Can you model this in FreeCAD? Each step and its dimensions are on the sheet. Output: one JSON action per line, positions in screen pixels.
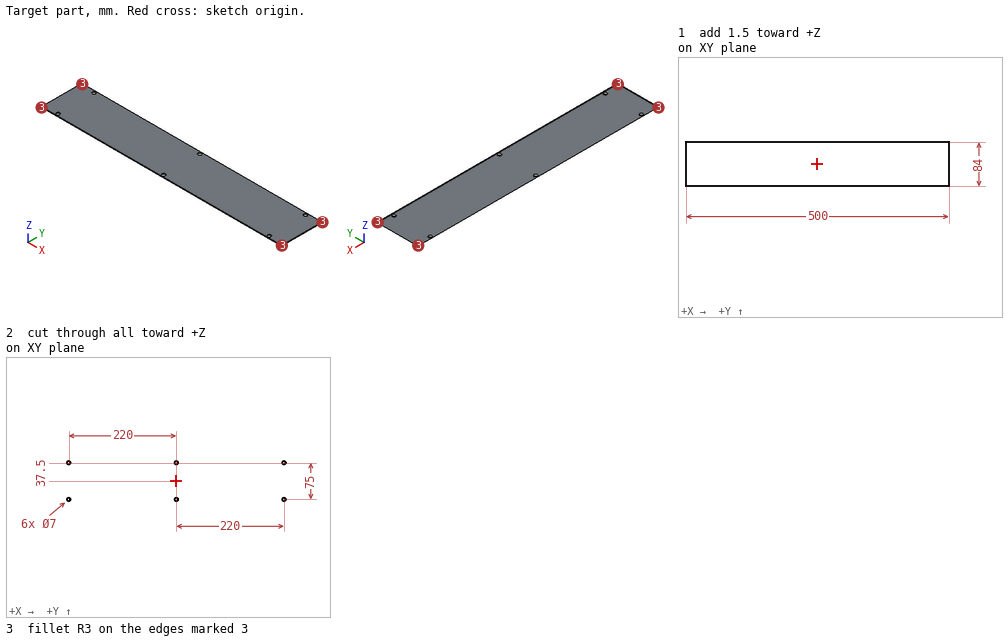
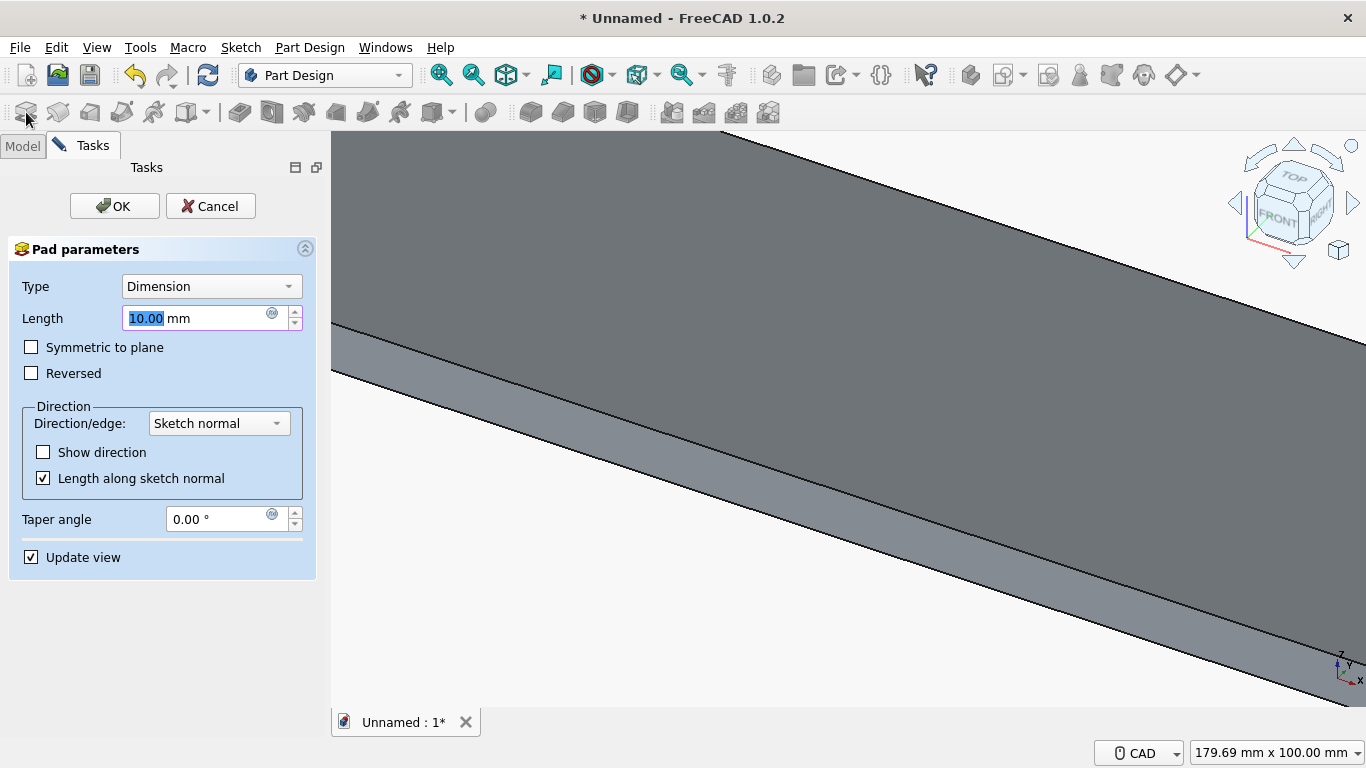
{"action": "type", "text": "1.5"}
{"action": "key", "text": "Tab"}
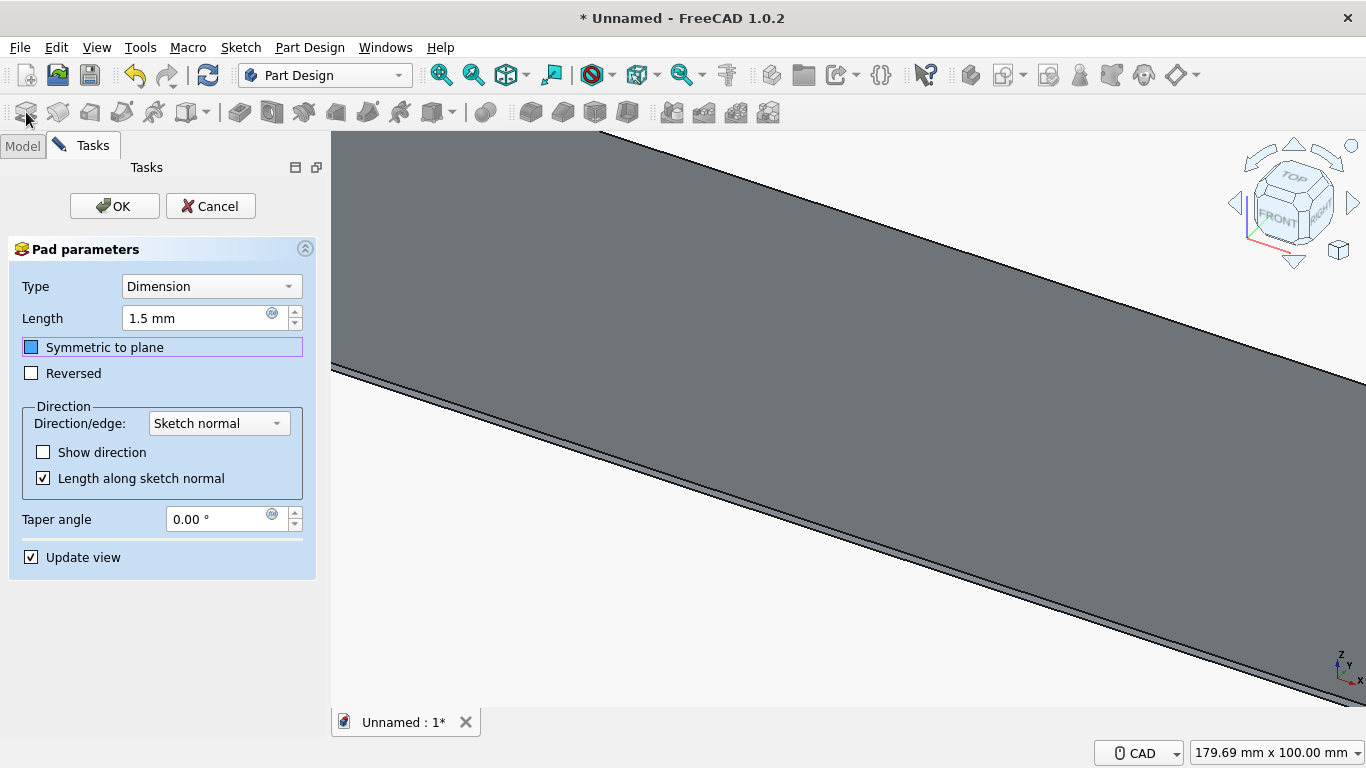
{"action": "left_click", "coordinate": [115, 206]}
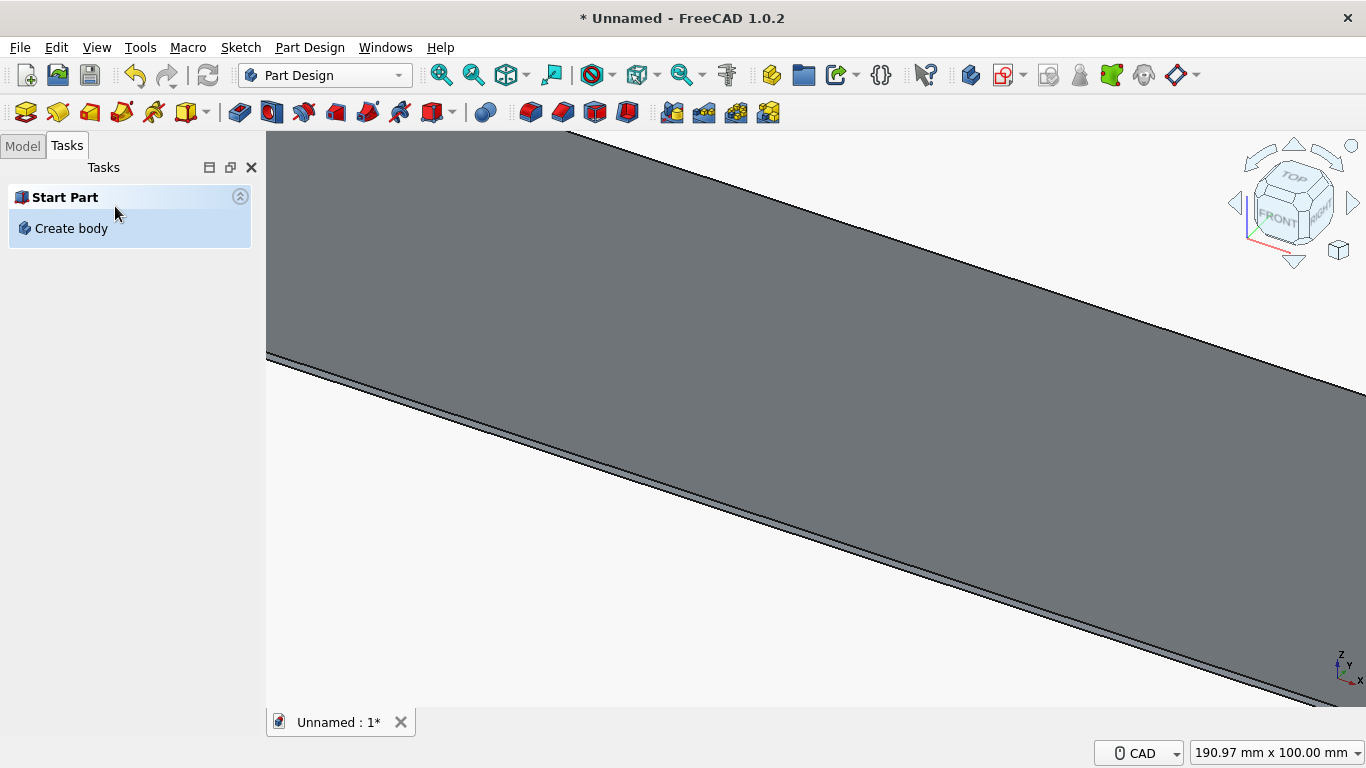
{"action": "left_click", "coordinate": [442, 76]}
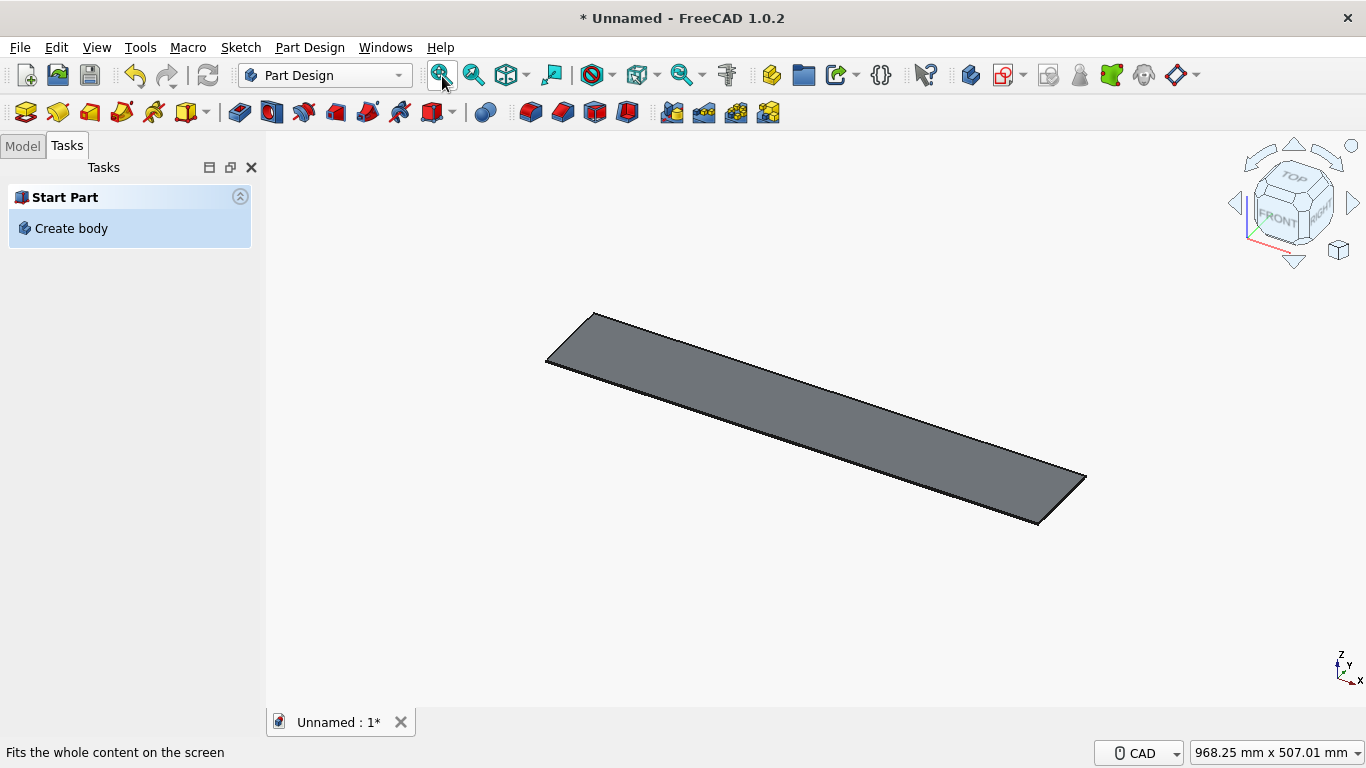
{"action": "left_click", "coordinate": [1004, 76]}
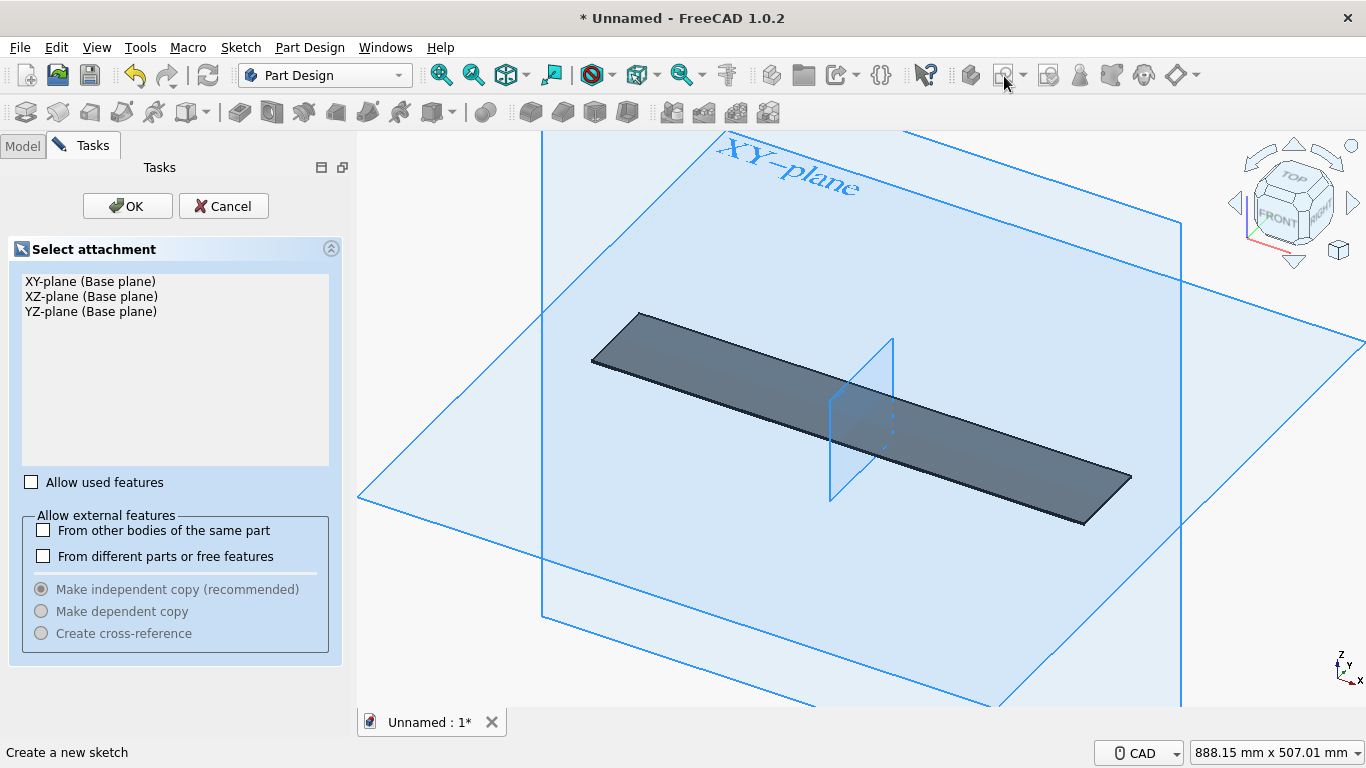
{"action": "left_click", "coordinate": [82, 282]}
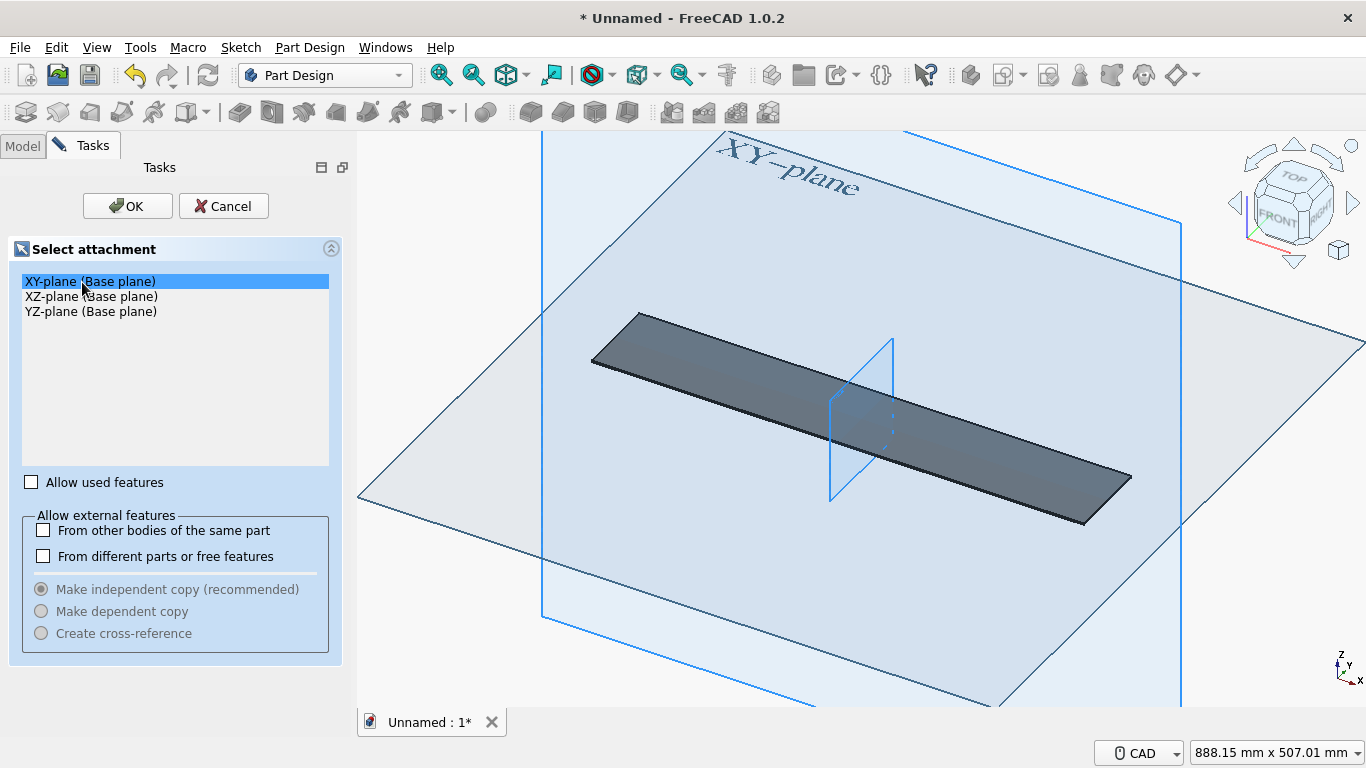
{"action": "left_click", "coordinate": [128, 206]}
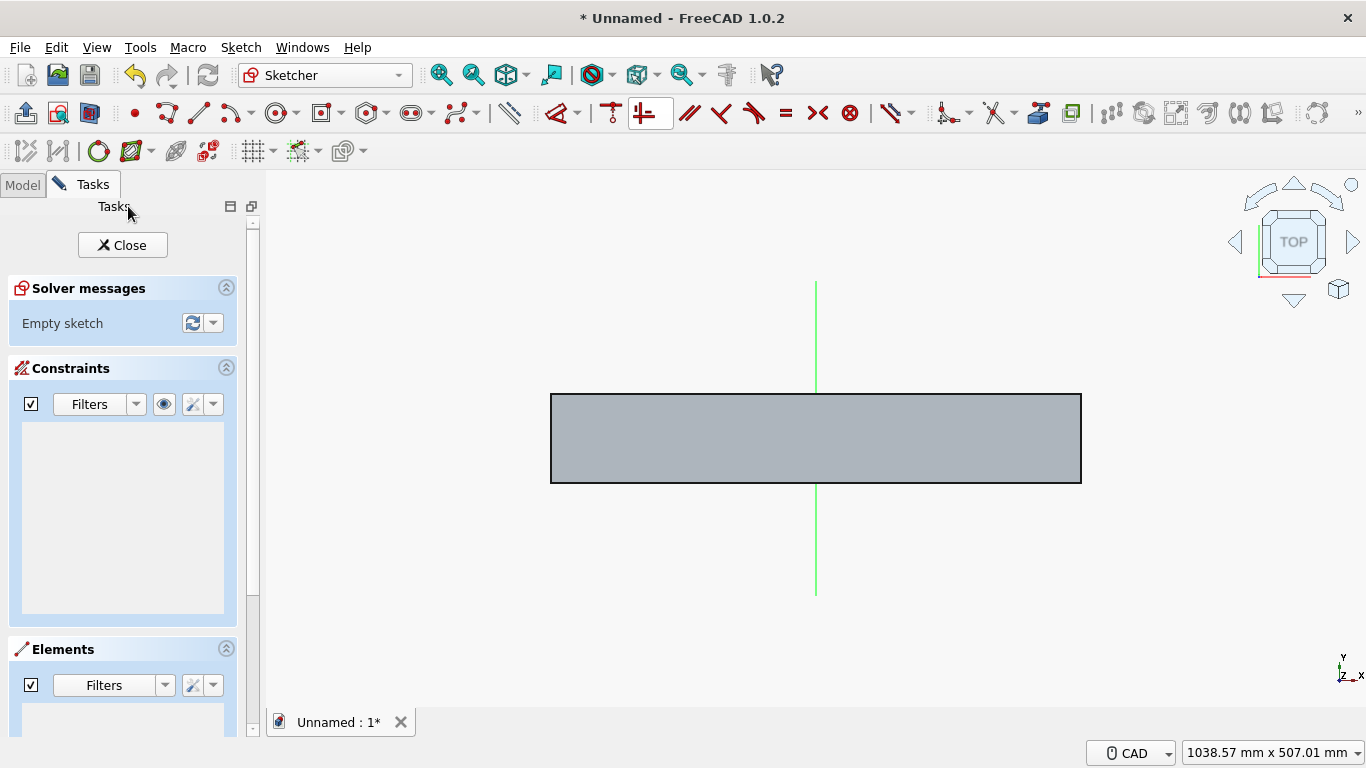
{"action": "left_click", "coordinate": [90, 114]}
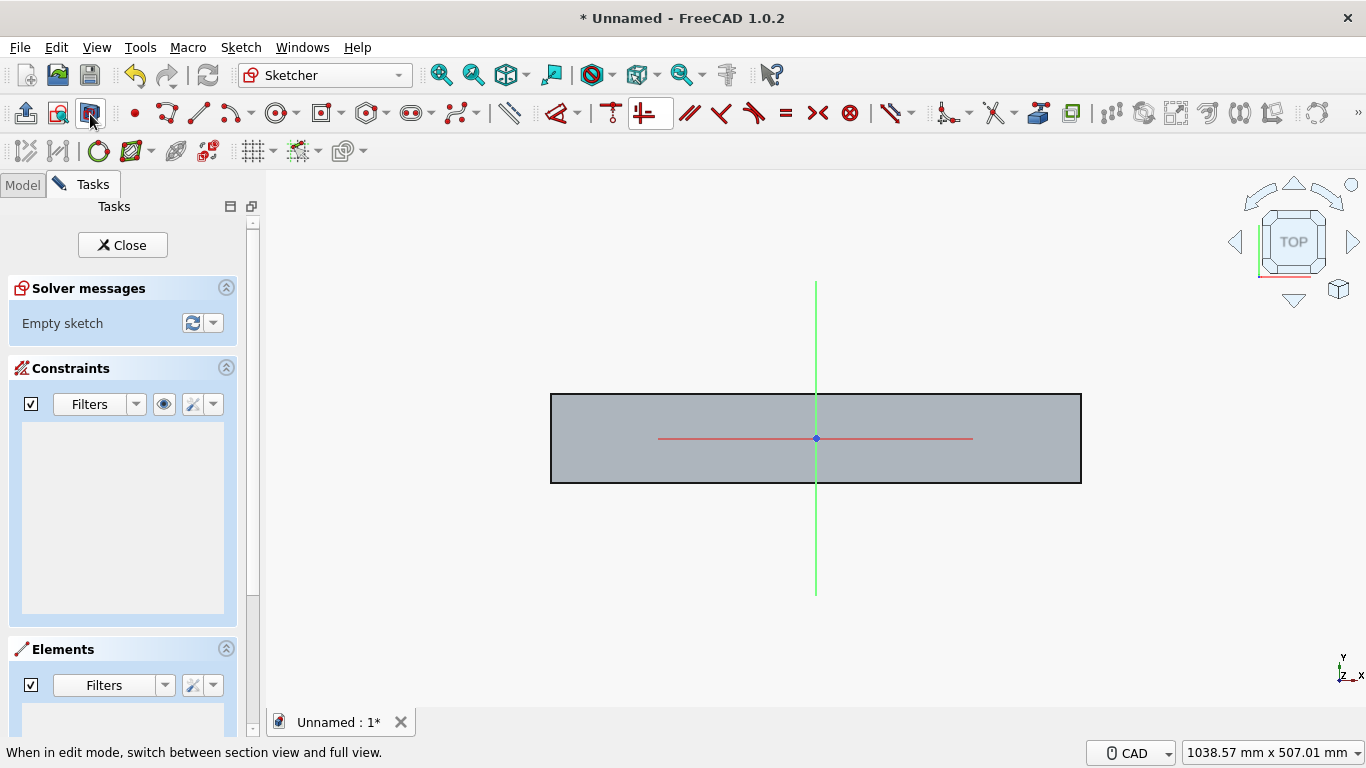
{"action": "scroll", "coordinate": [955, 439], "scroll_direction": "up", "scroll_amount": 2}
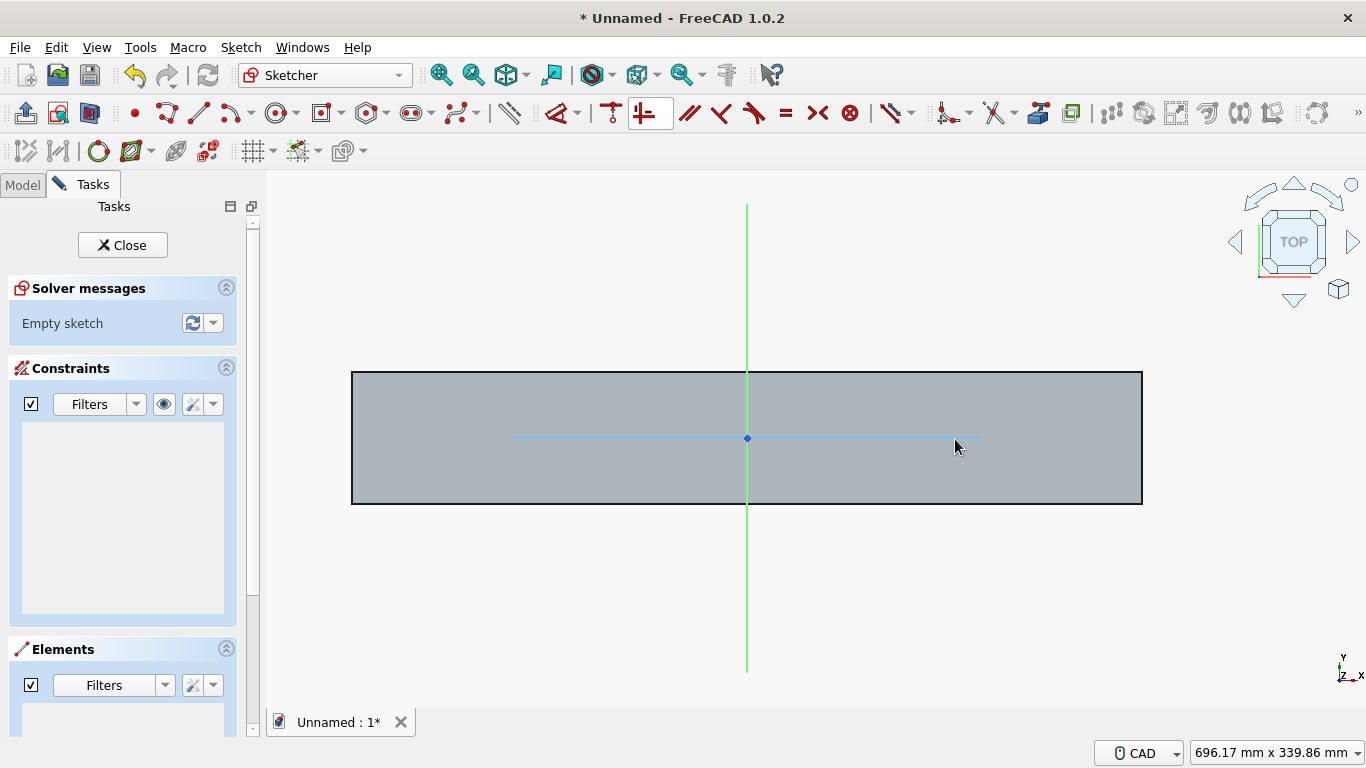
{"action": "left_click", "coordinate": [276, 114]}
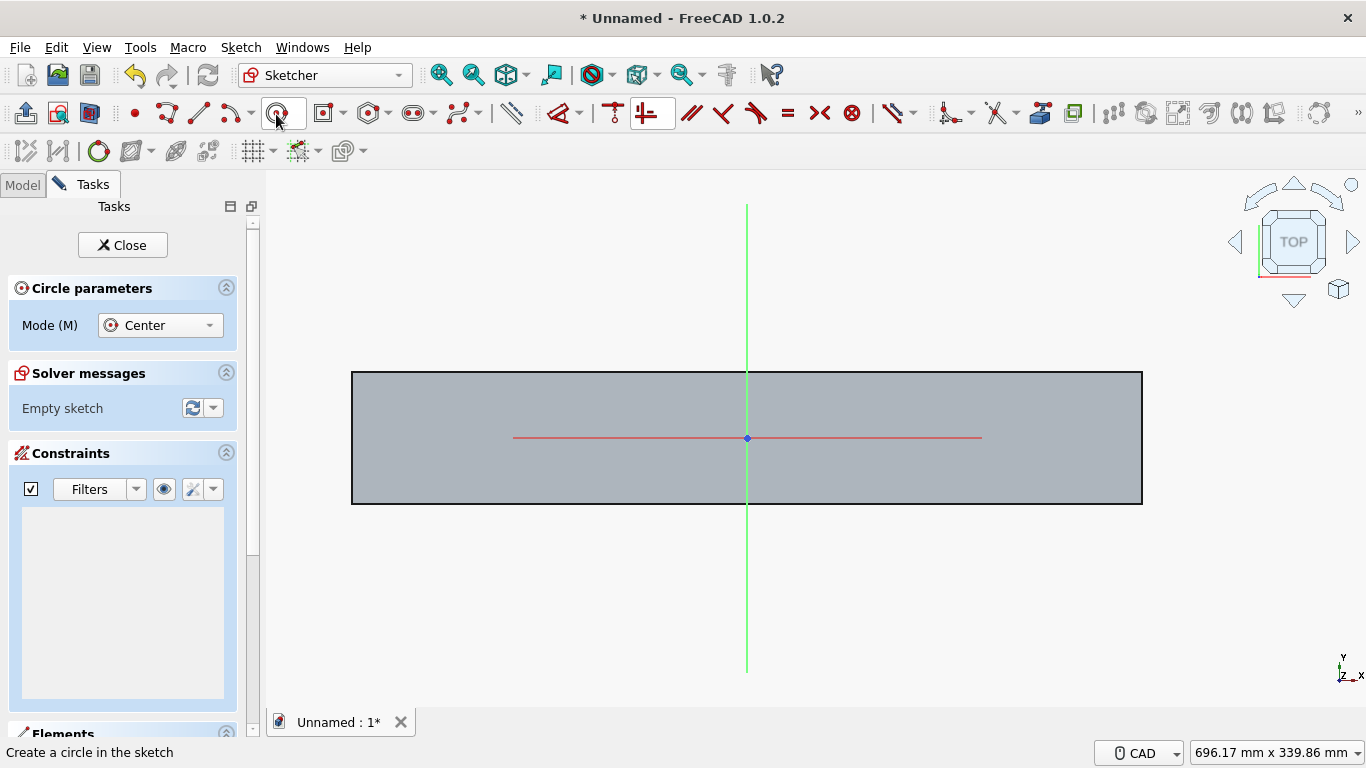
{"action": "scroll", "coordinate": [747, 379], "scroll_direction": "up", "scroll_amount": 8}